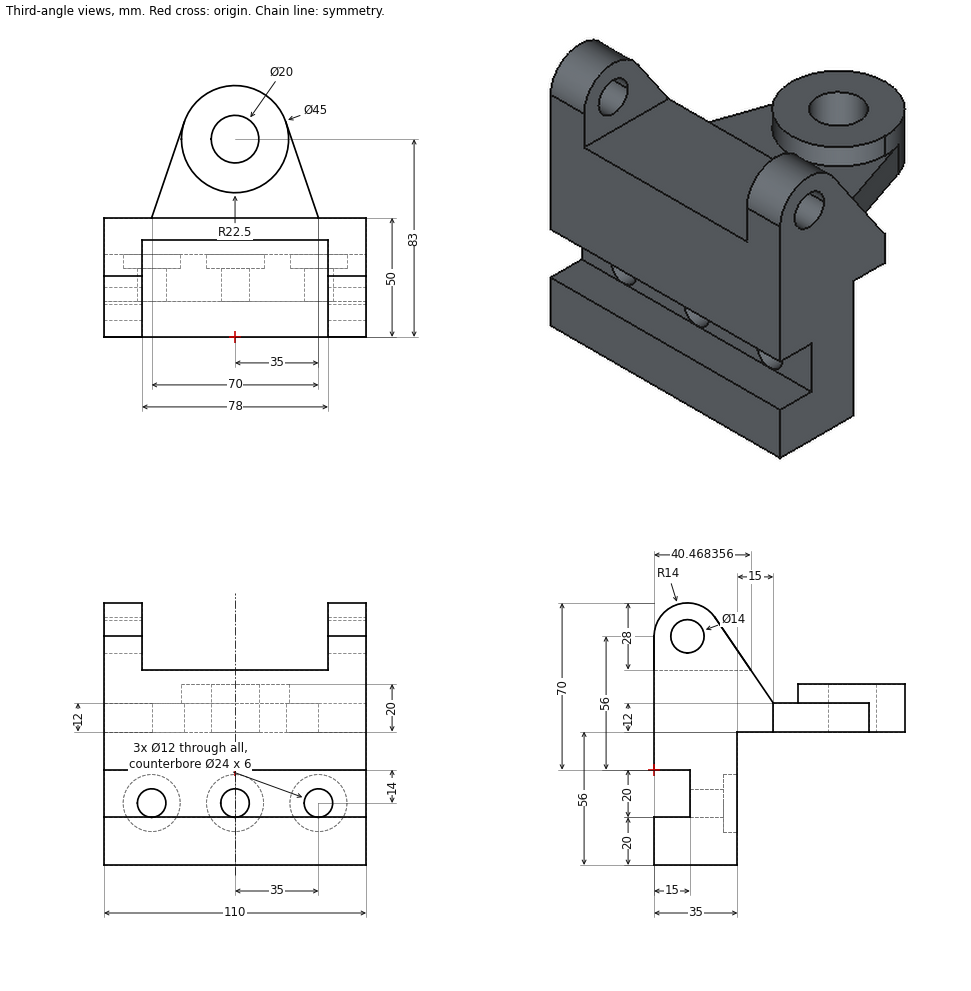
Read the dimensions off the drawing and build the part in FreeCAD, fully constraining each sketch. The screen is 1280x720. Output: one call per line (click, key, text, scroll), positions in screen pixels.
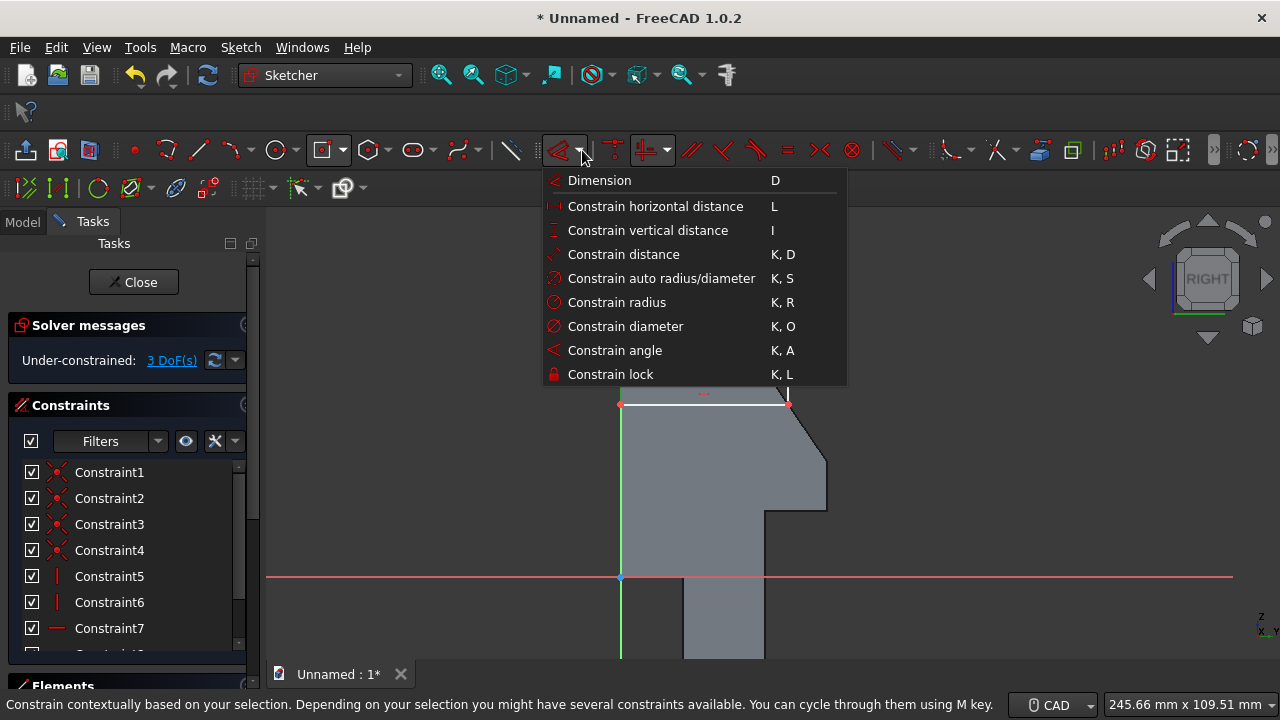
click(695, 230)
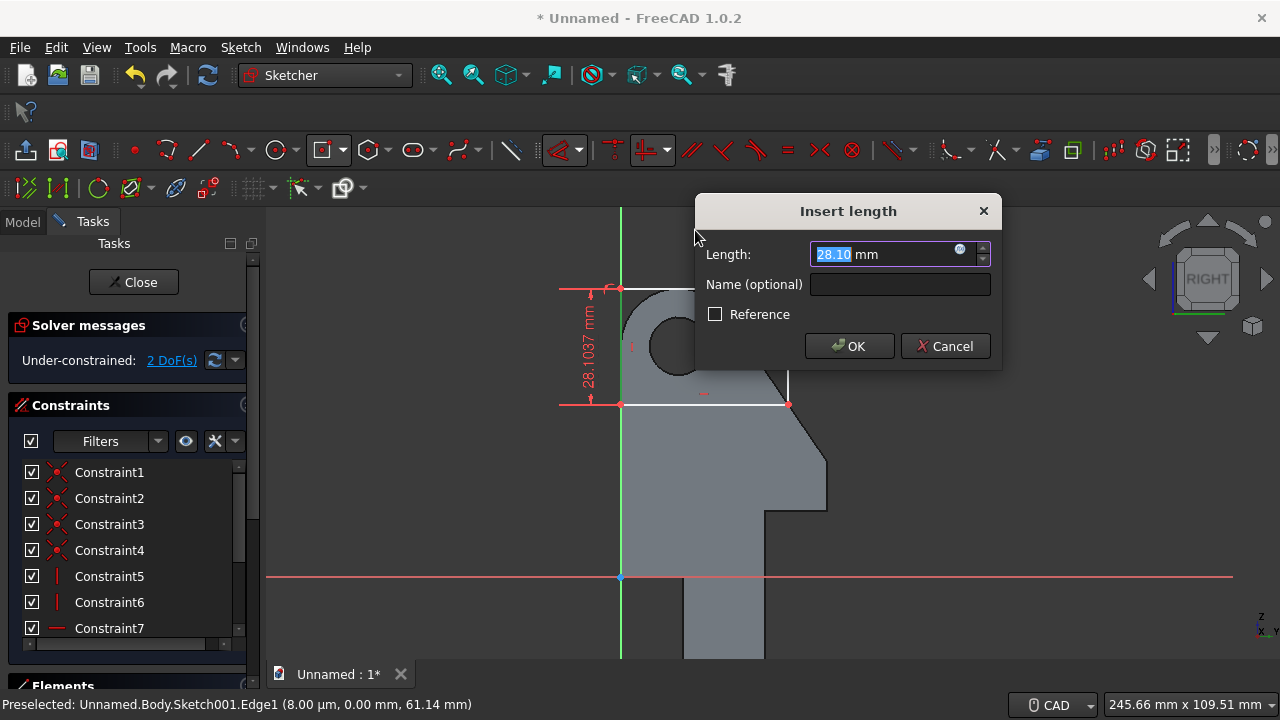
text(28)
key(Return)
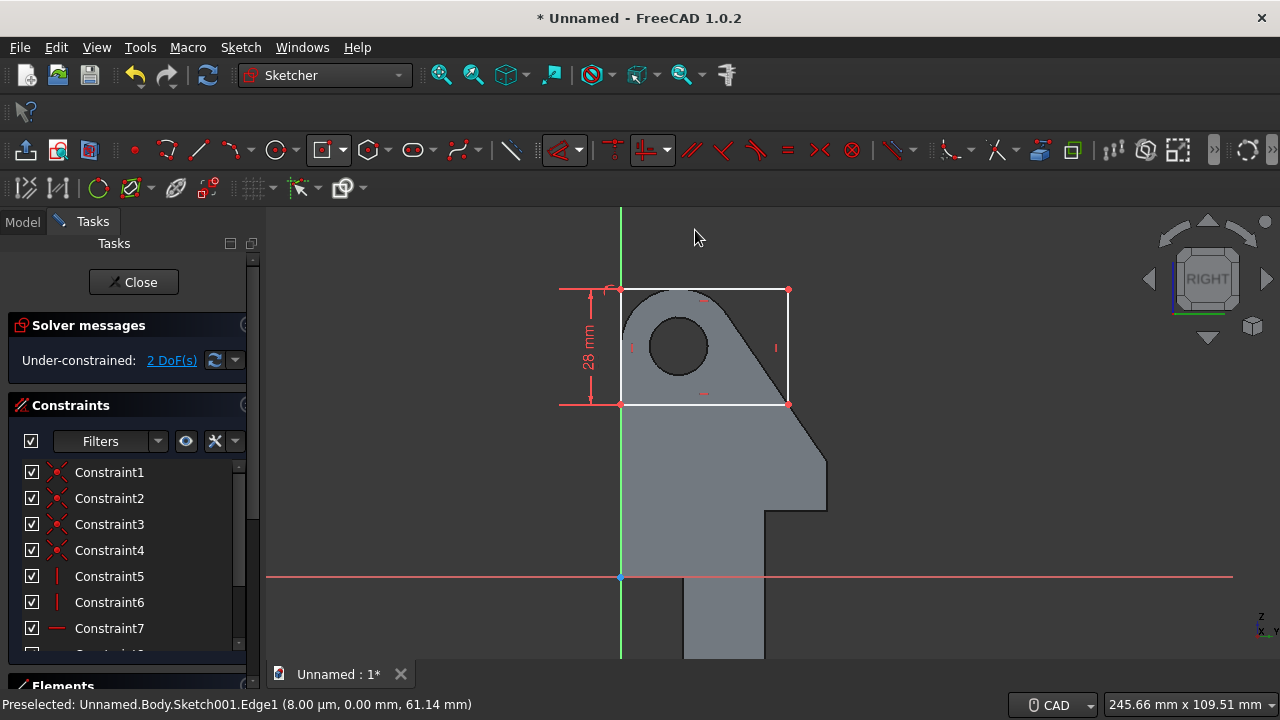
click(621, 289)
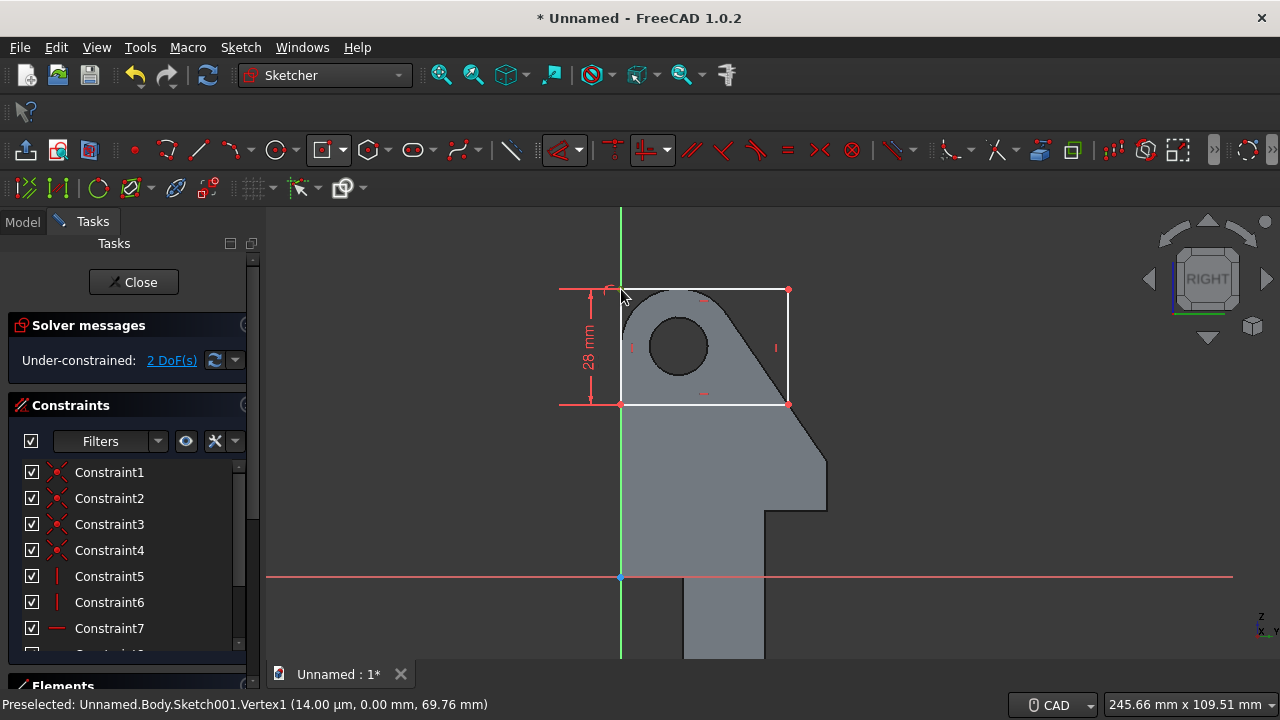
click(582, 150)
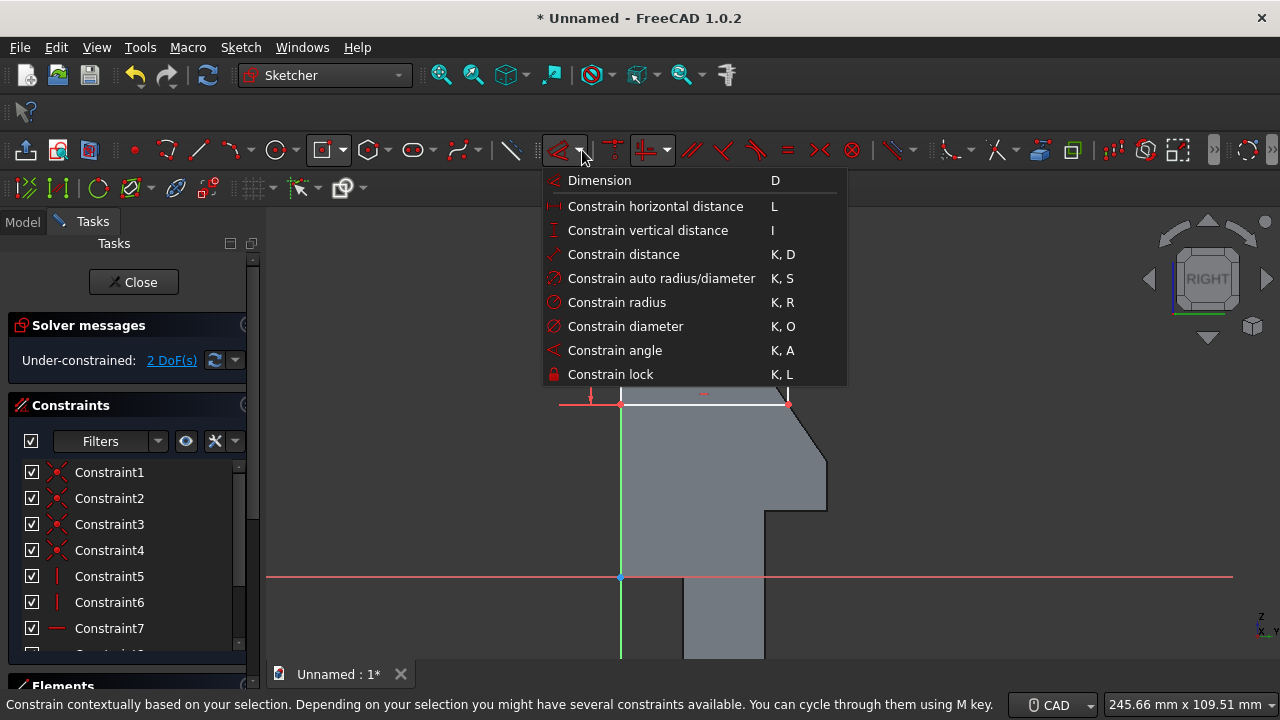
click(695, 230)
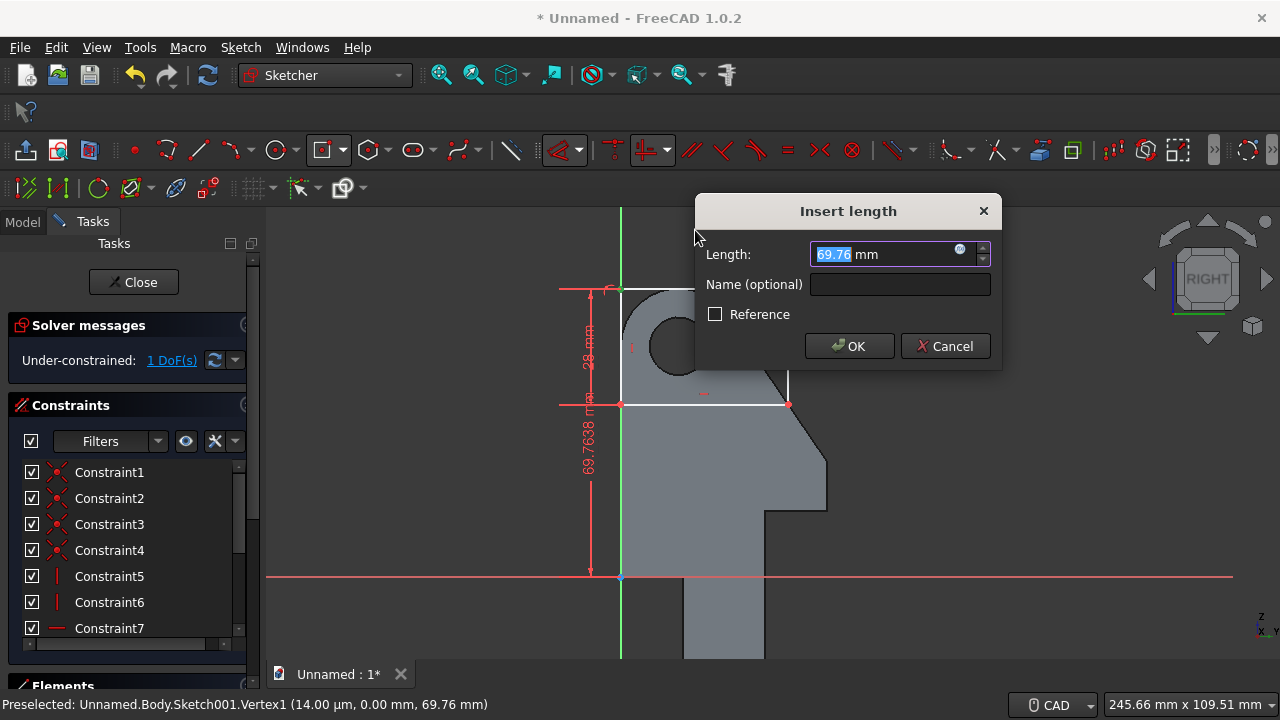
text(70)
key(Return)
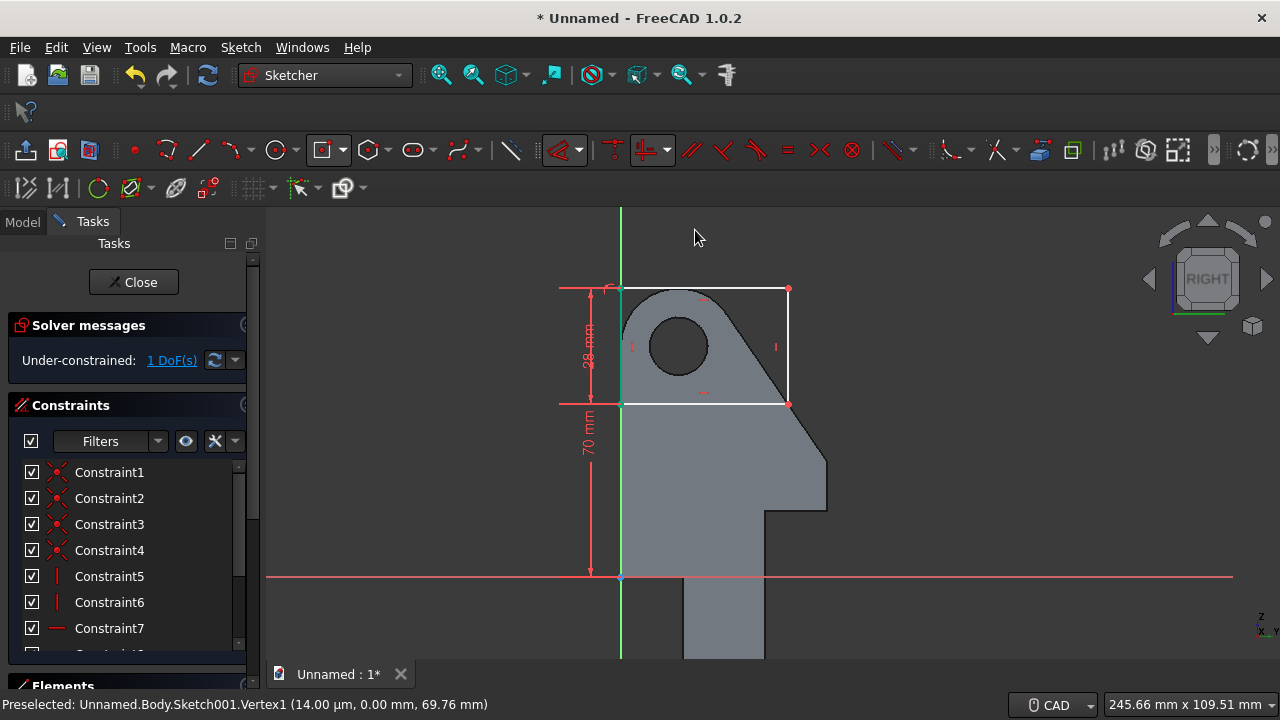
click(671, 404)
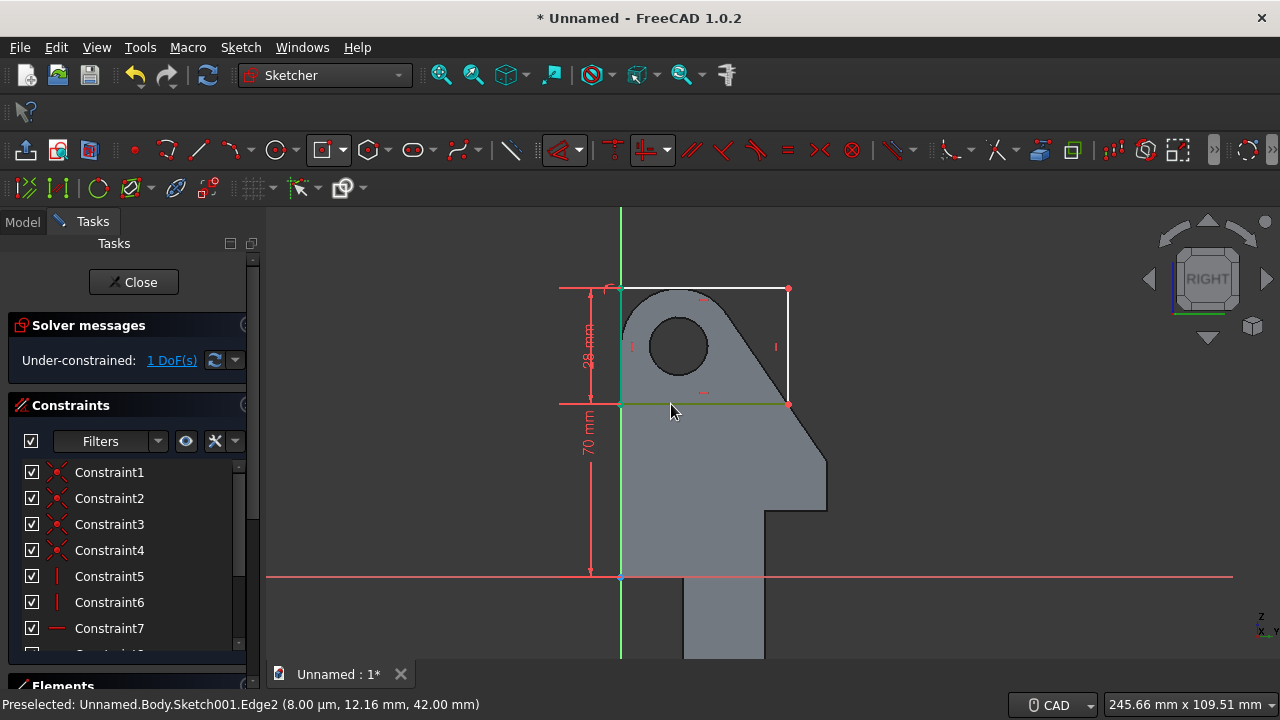
key(l)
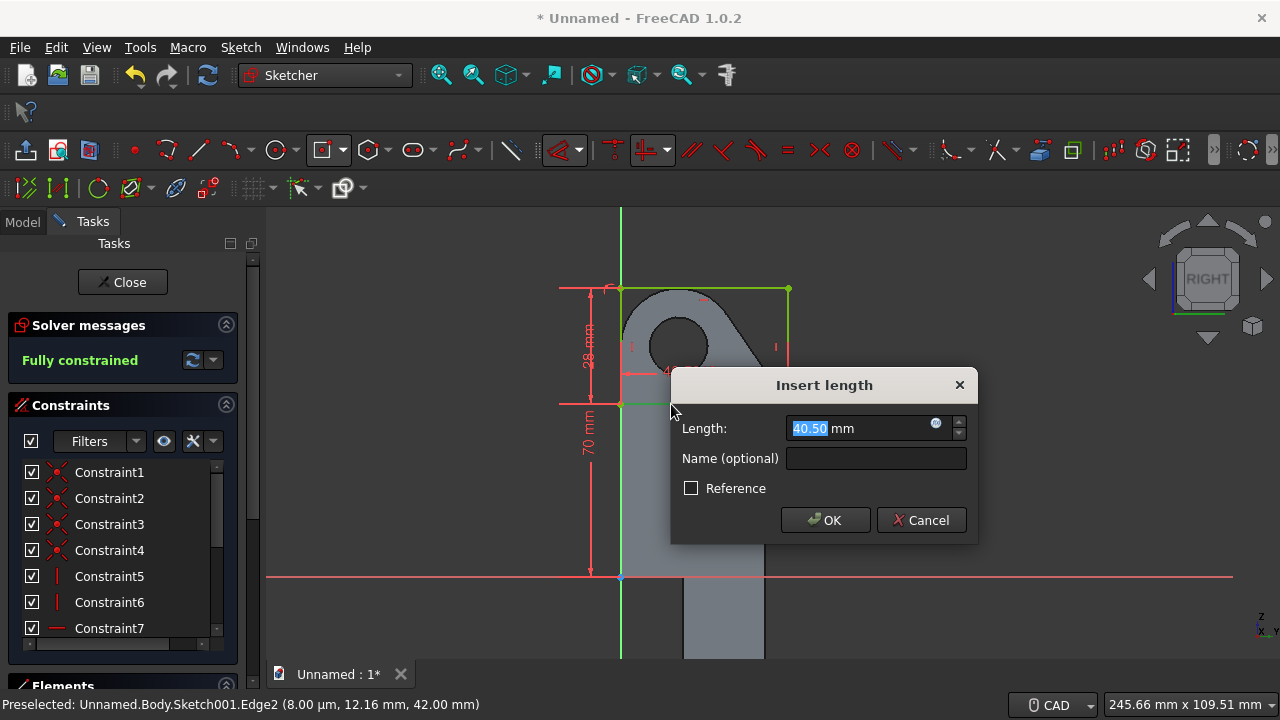
text(40.468356)
key(Return)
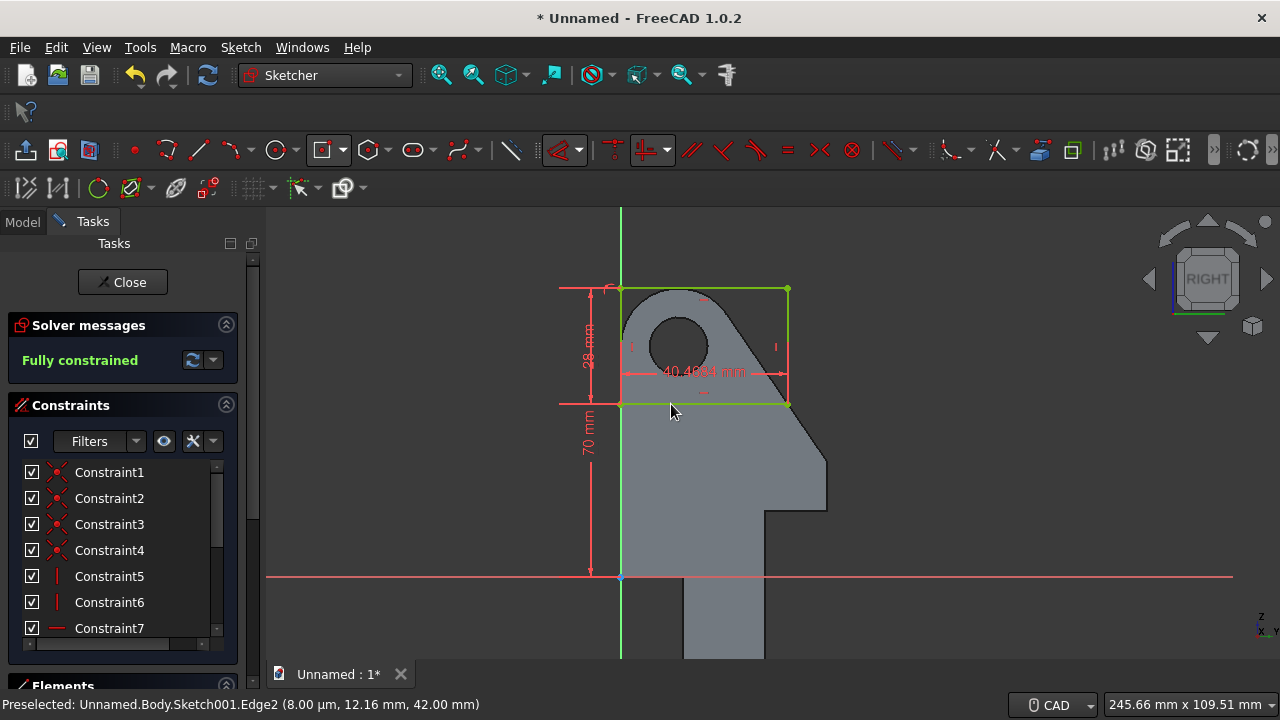
click(123, 282)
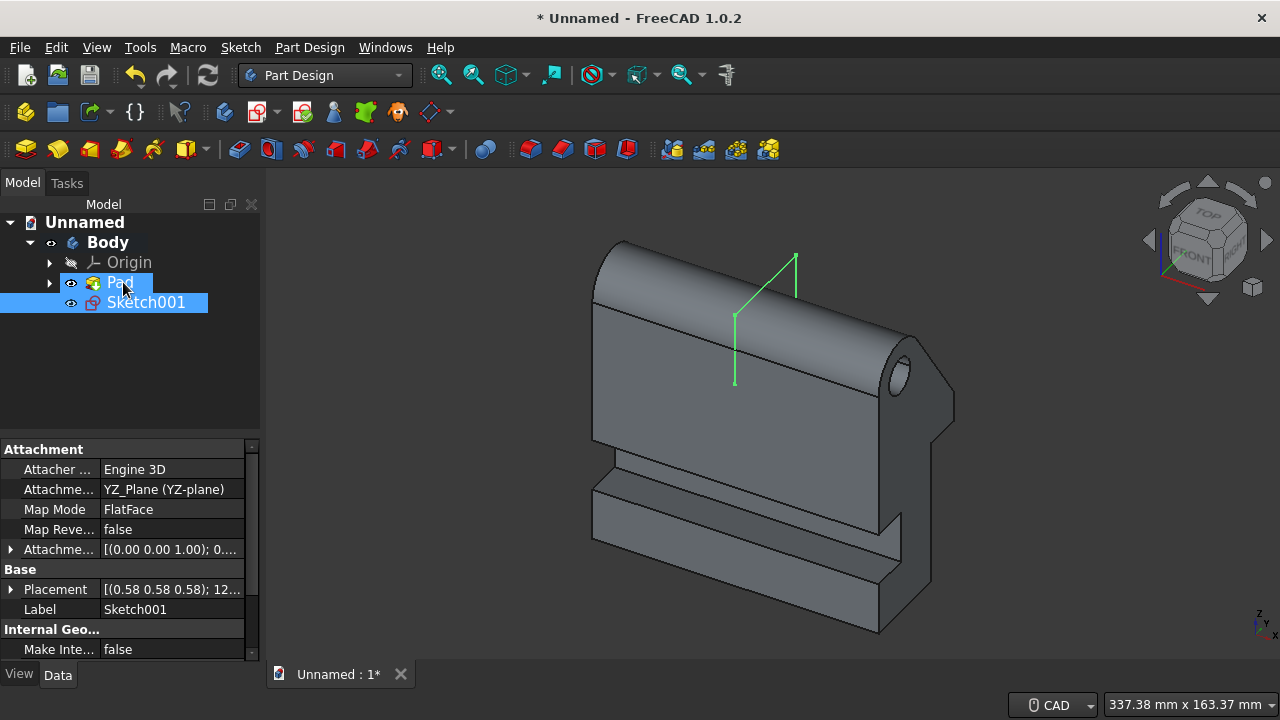
click(240, 150)